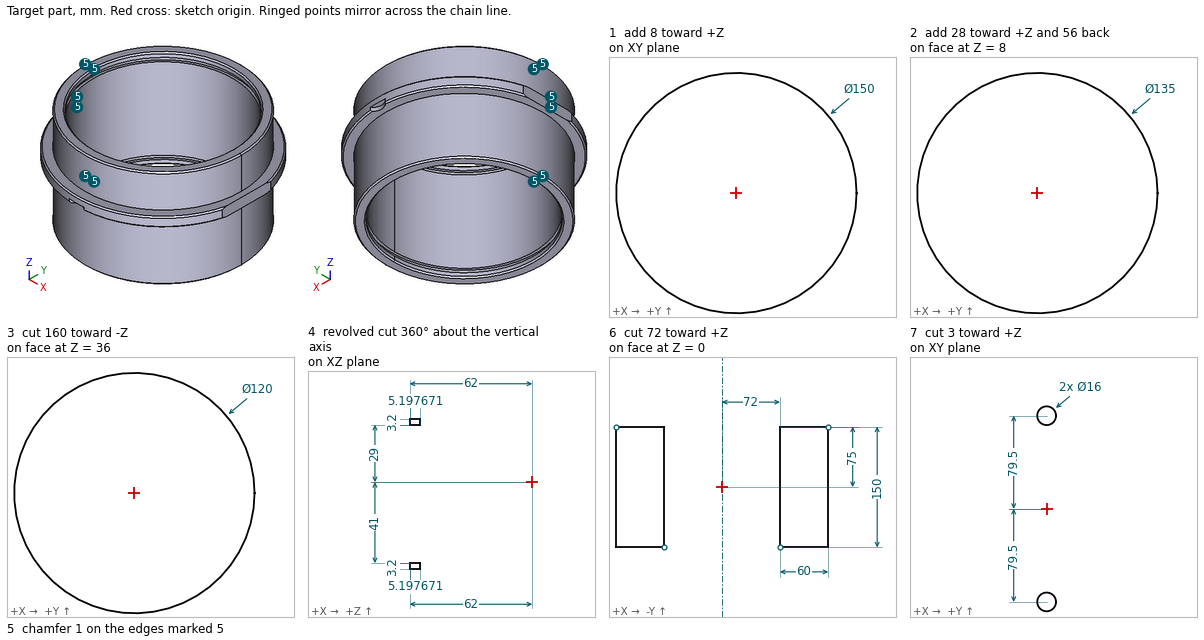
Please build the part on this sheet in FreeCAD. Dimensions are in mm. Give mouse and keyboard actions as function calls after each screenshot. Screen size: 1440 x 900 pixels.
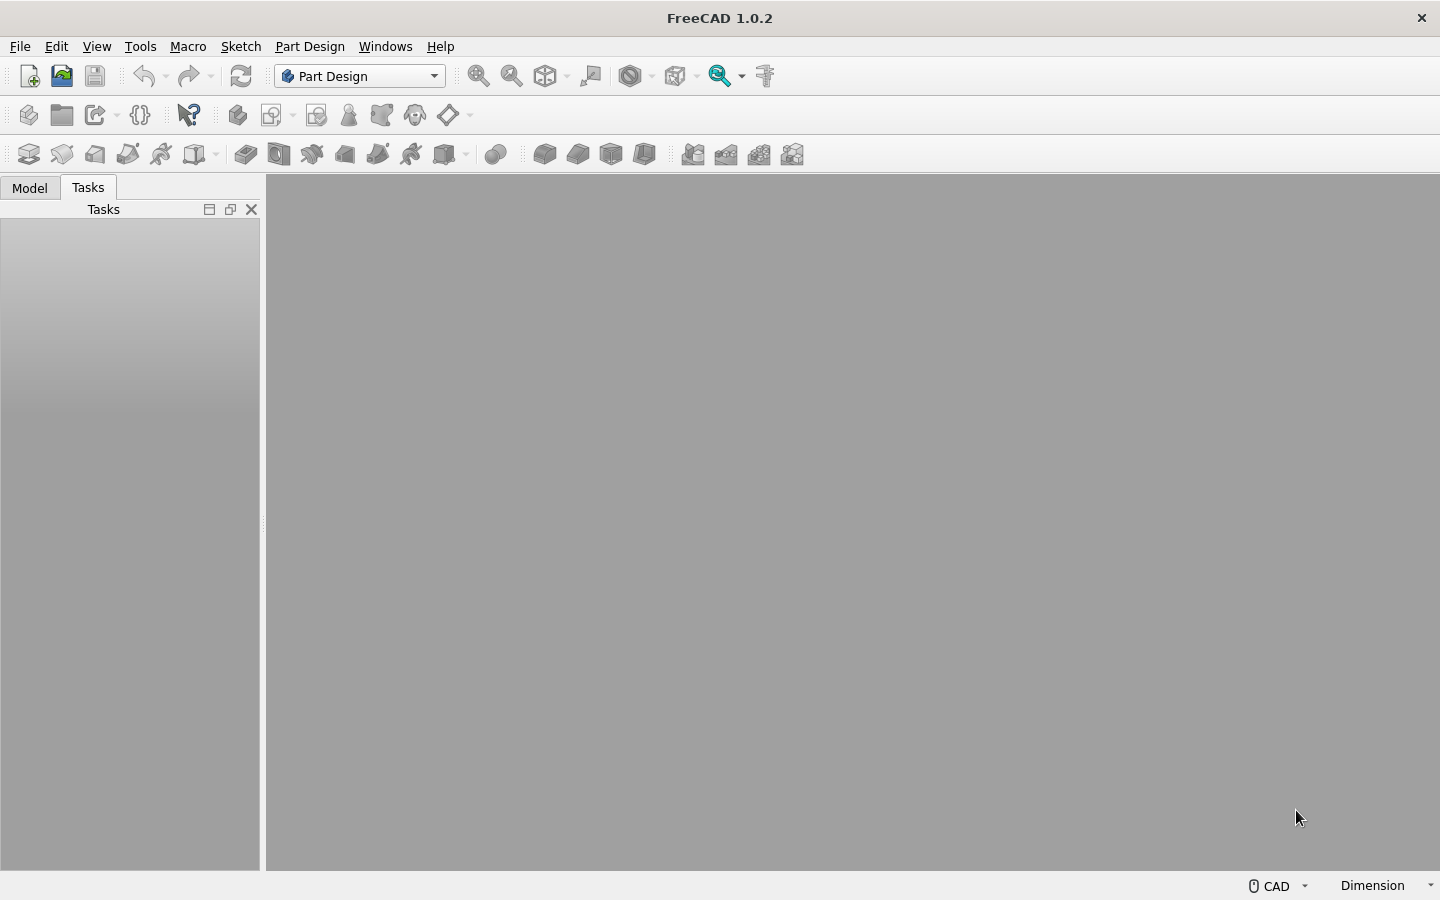
click(29, 76)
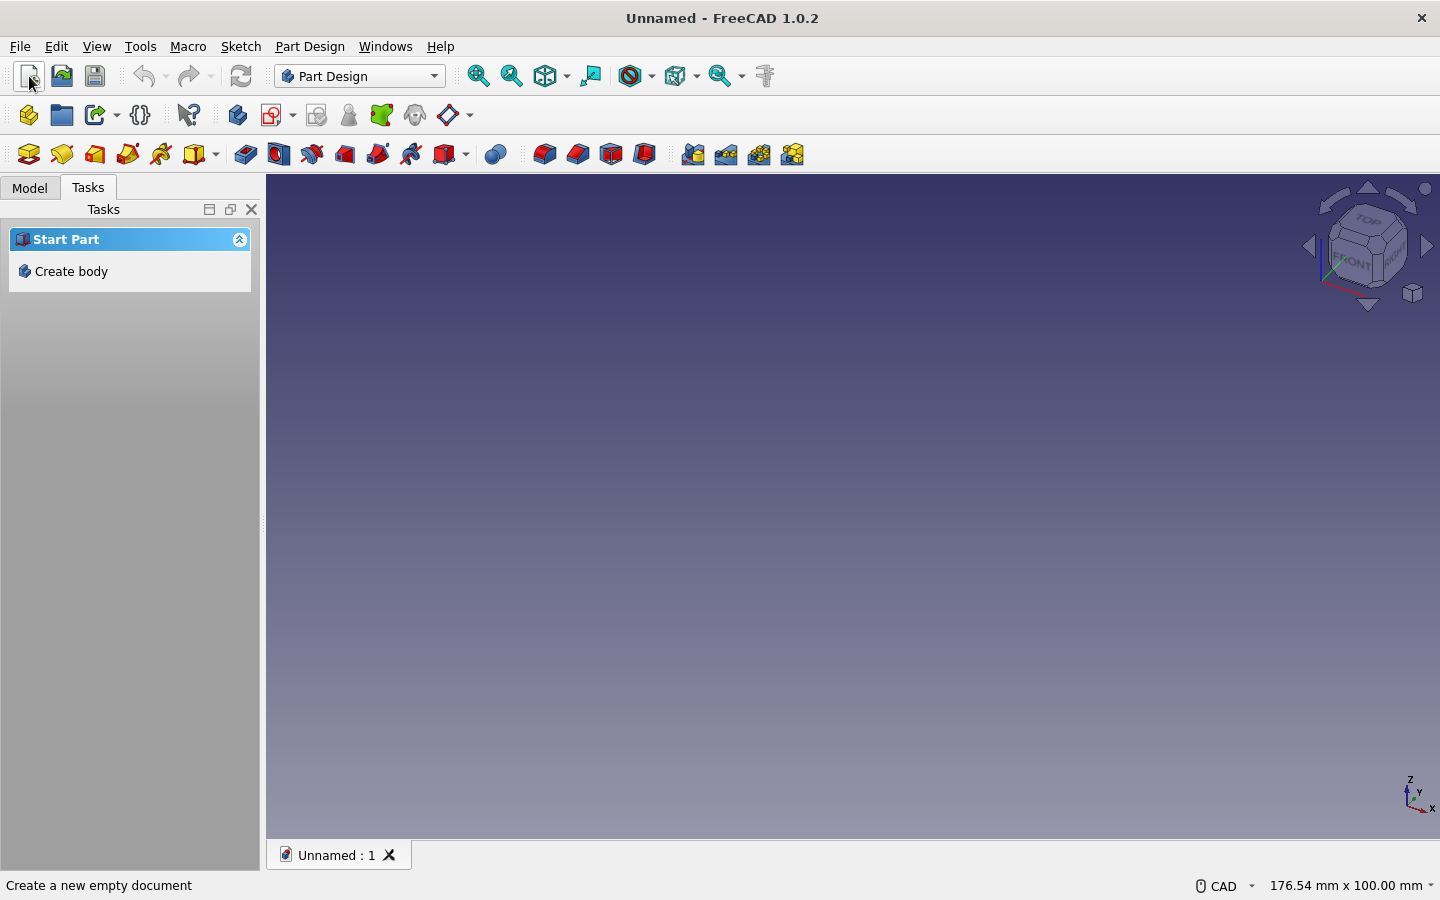
click(270, 116)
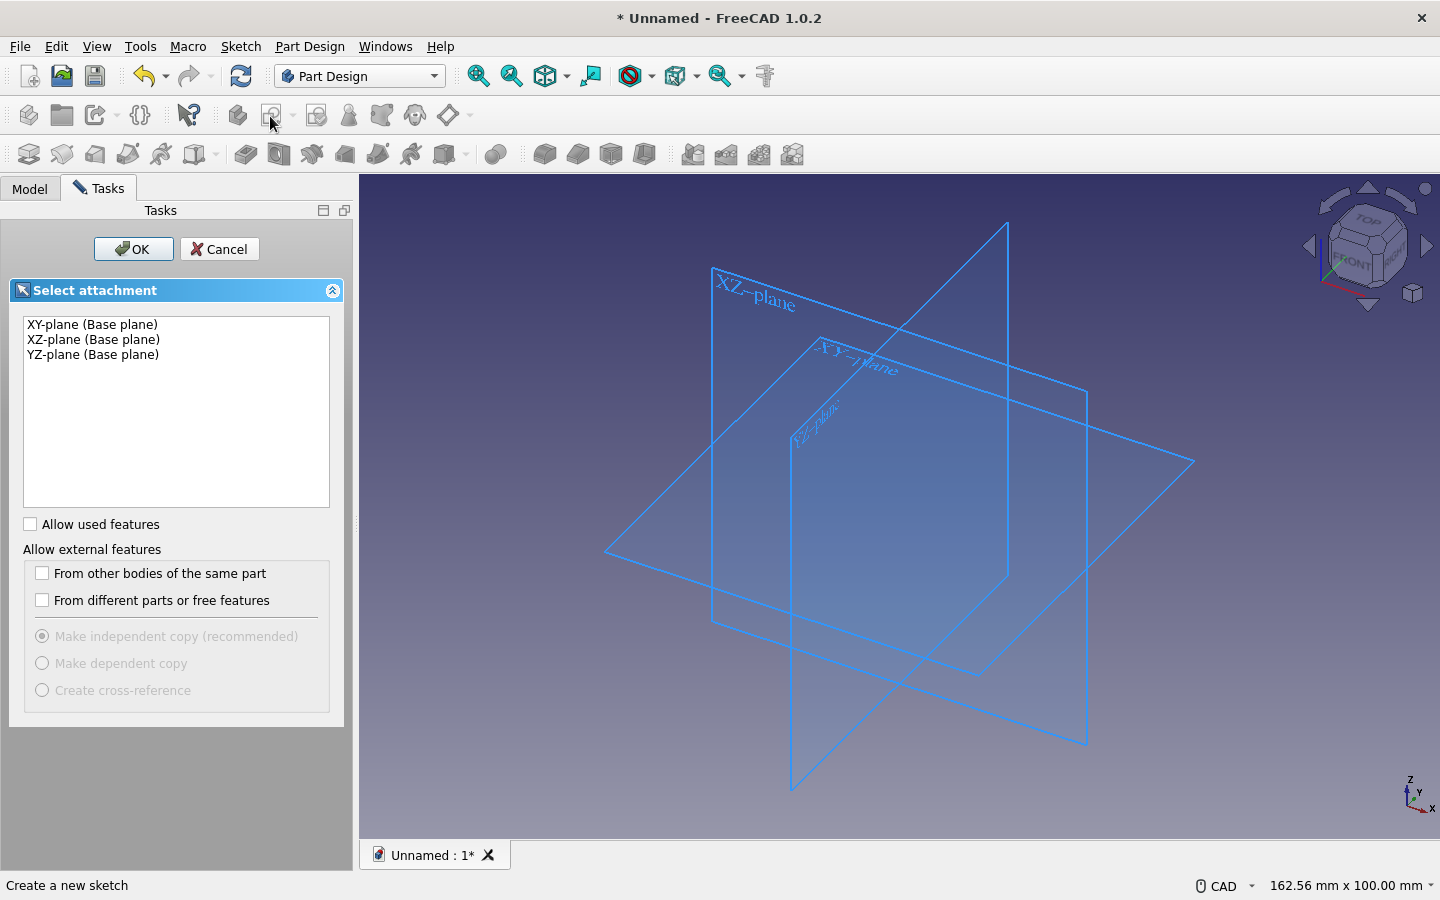
click(84, 324)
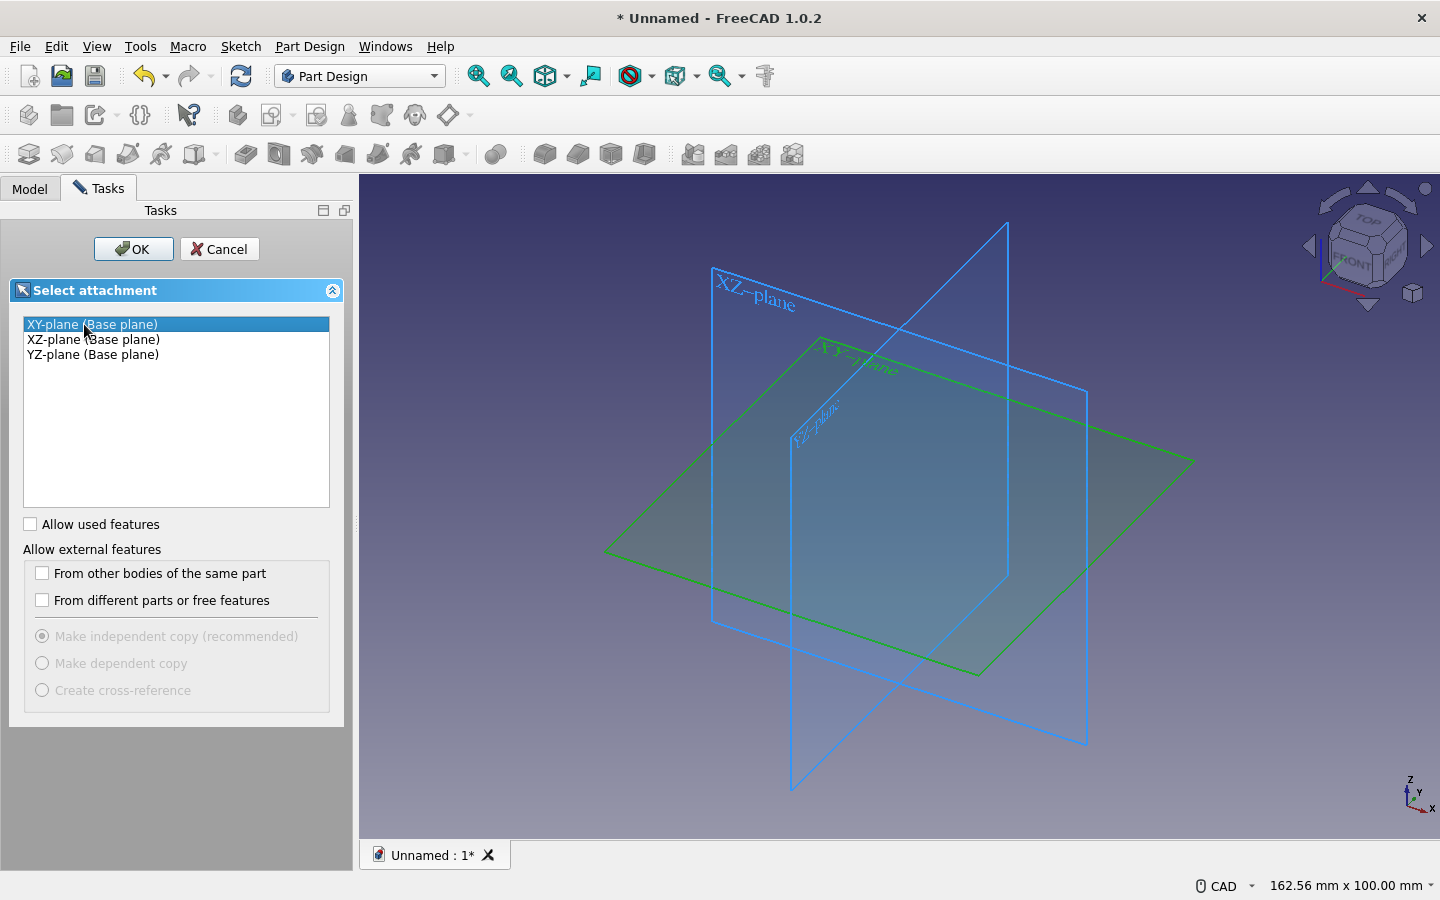
click(134, 249)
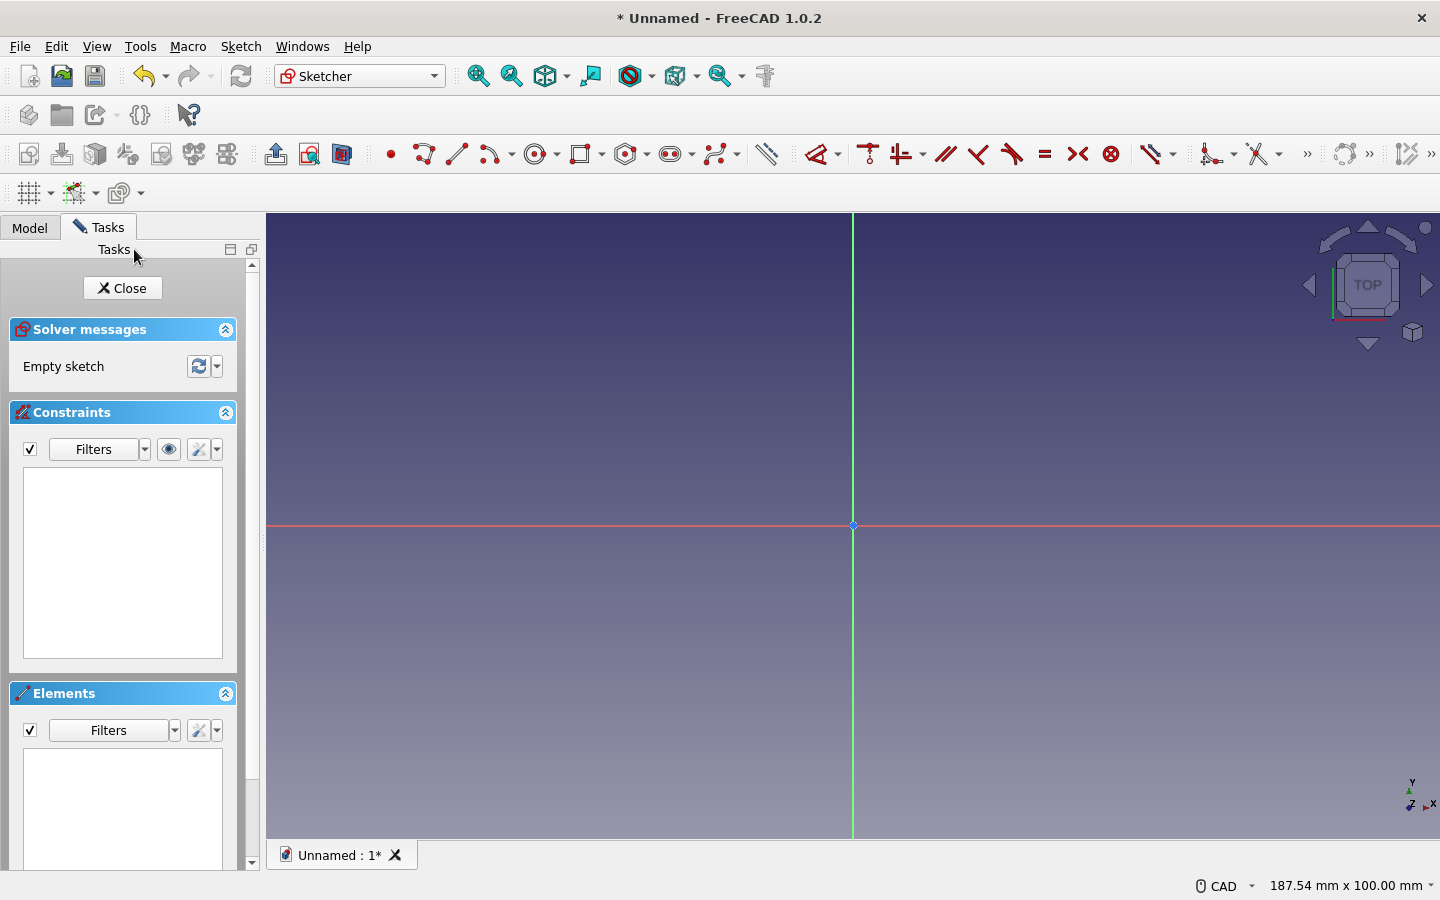
scroll(729, 526, down, 4)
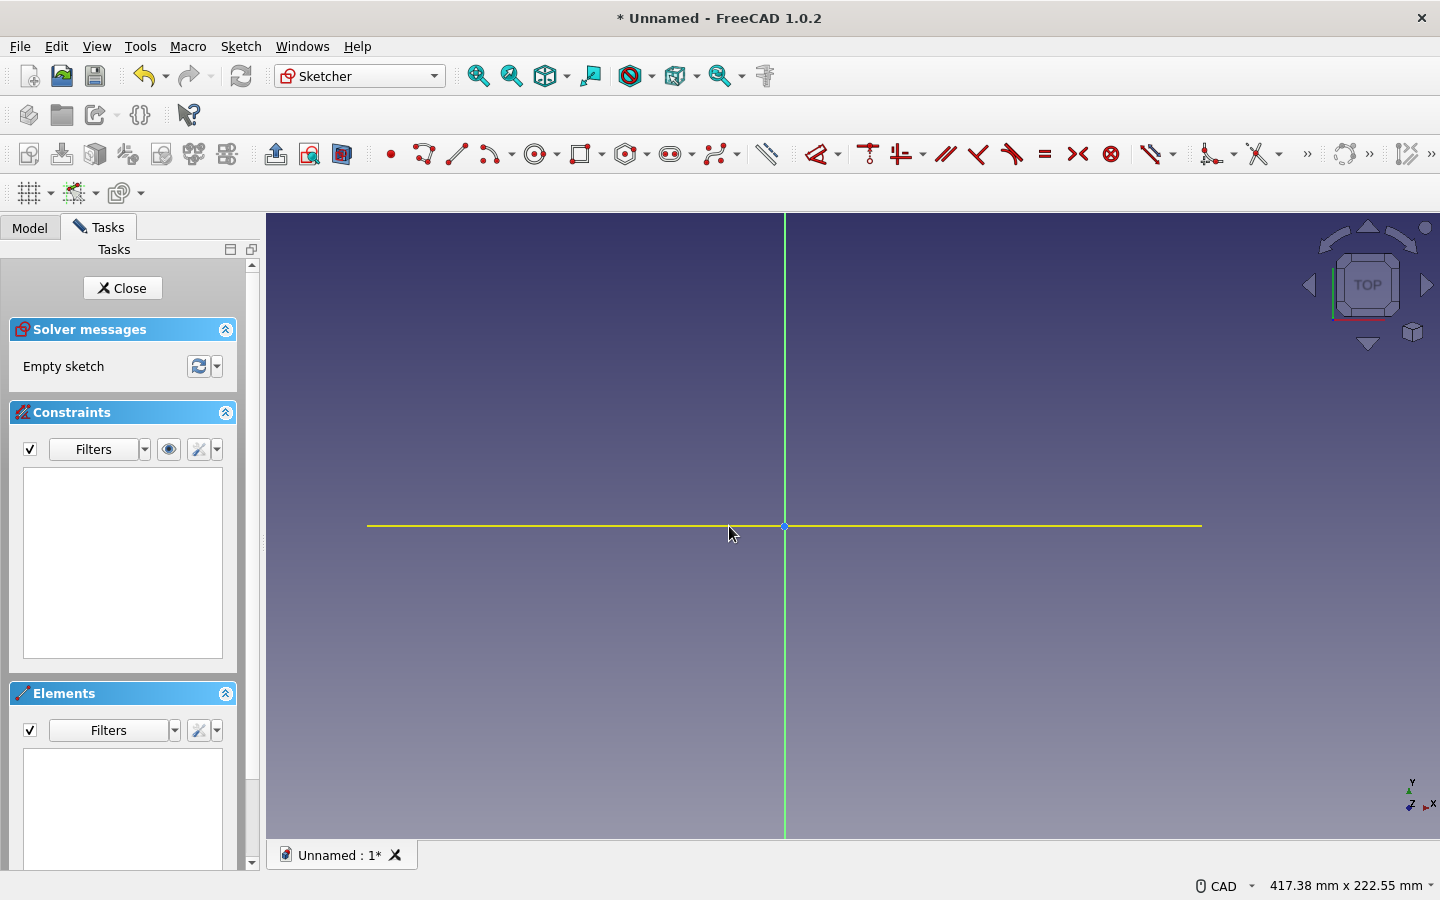
key(g)
key(c)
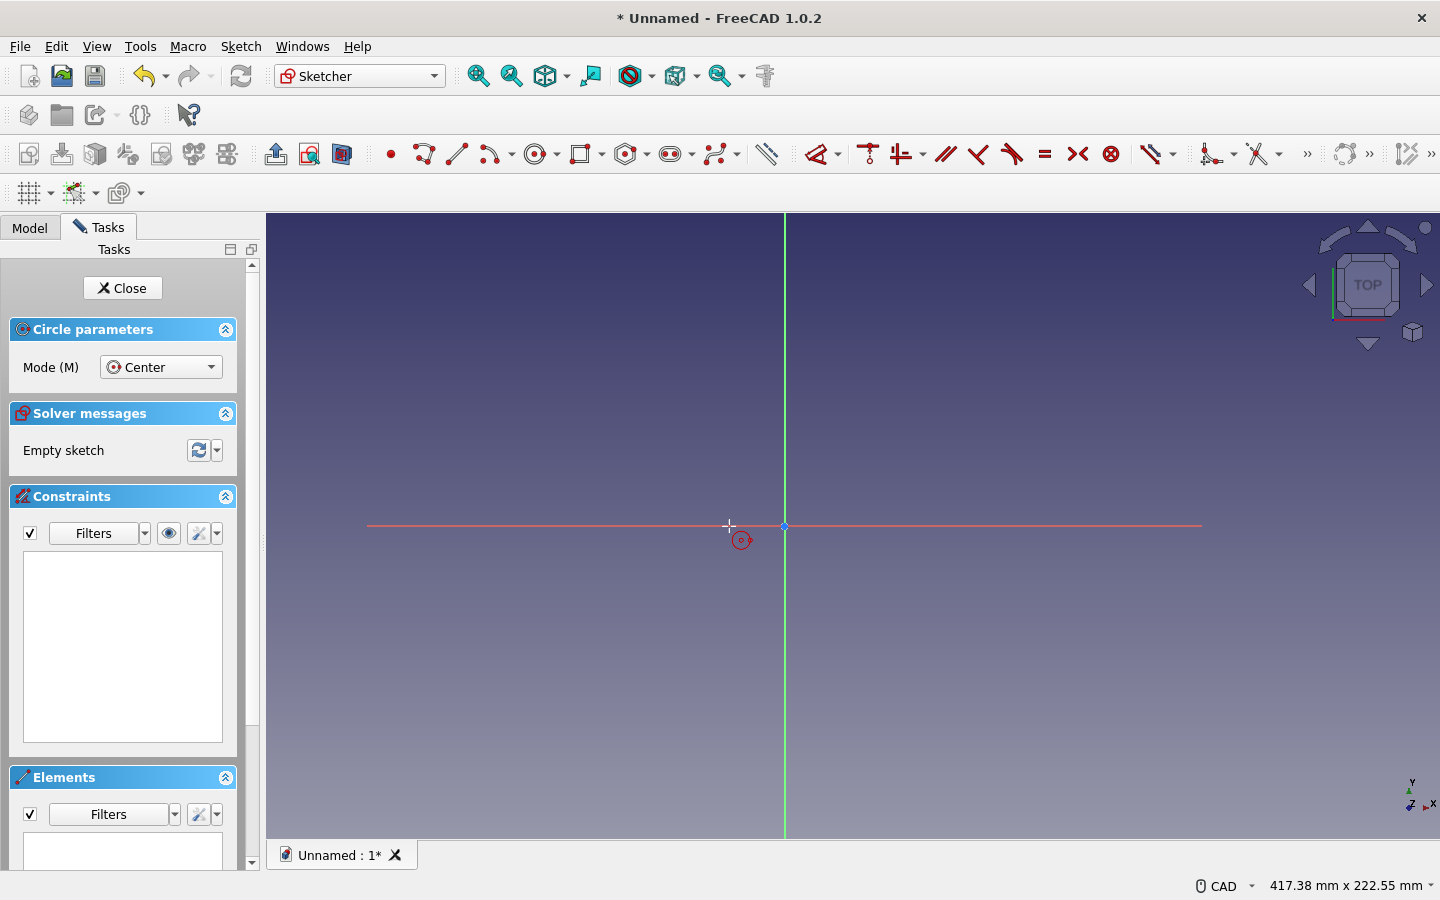
click(785, 526)
click(934, 377)
key(Escape)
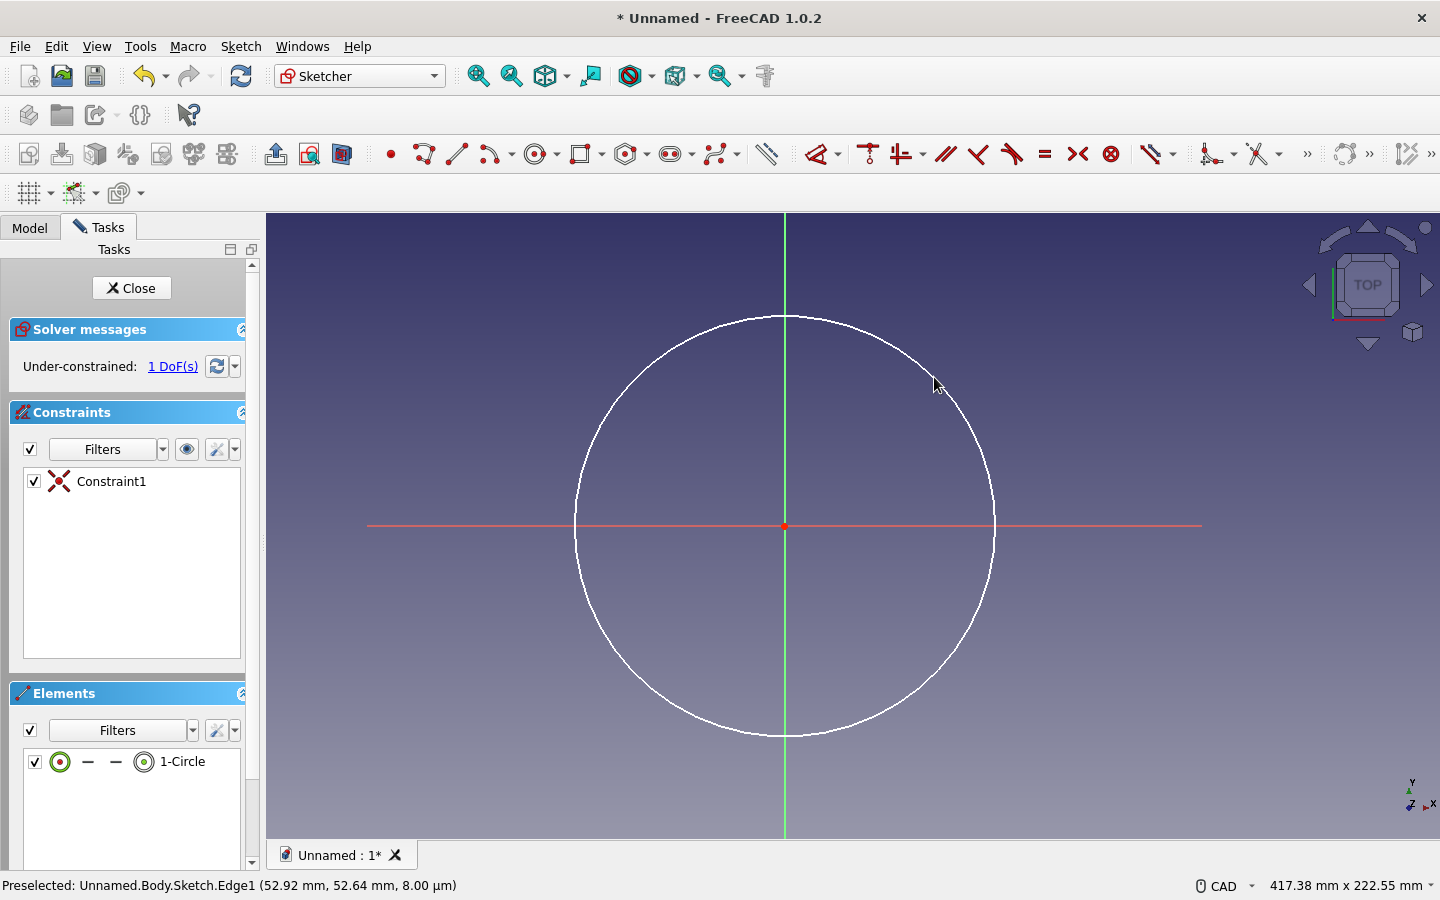
key(d)